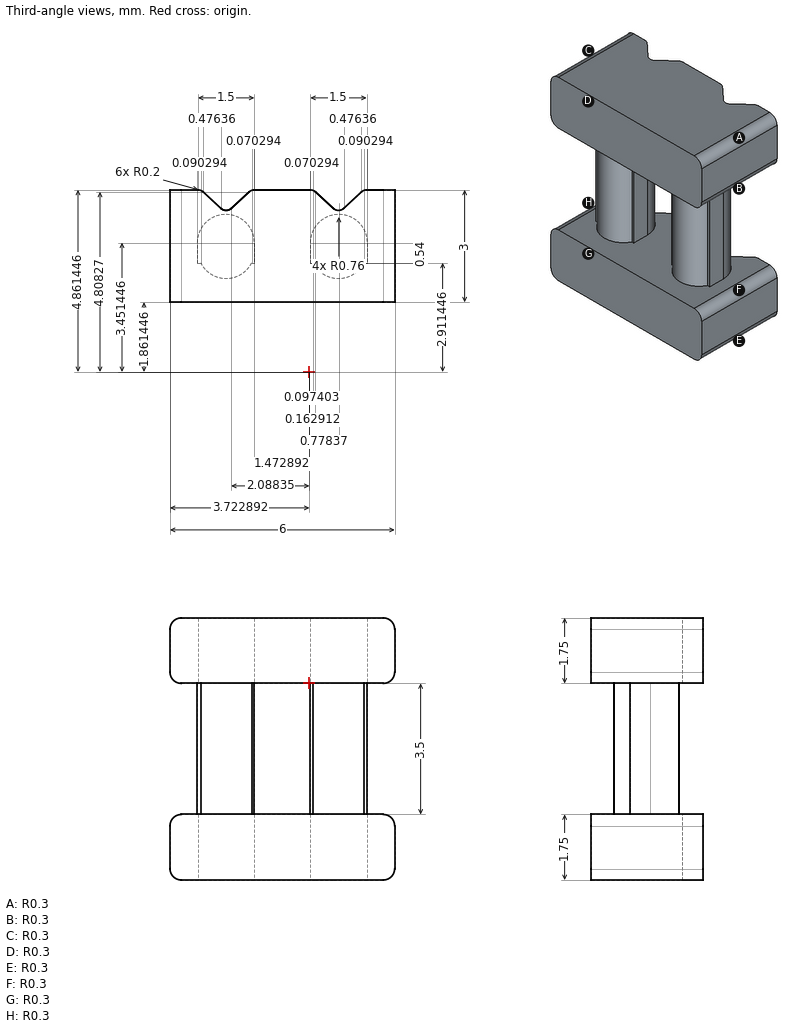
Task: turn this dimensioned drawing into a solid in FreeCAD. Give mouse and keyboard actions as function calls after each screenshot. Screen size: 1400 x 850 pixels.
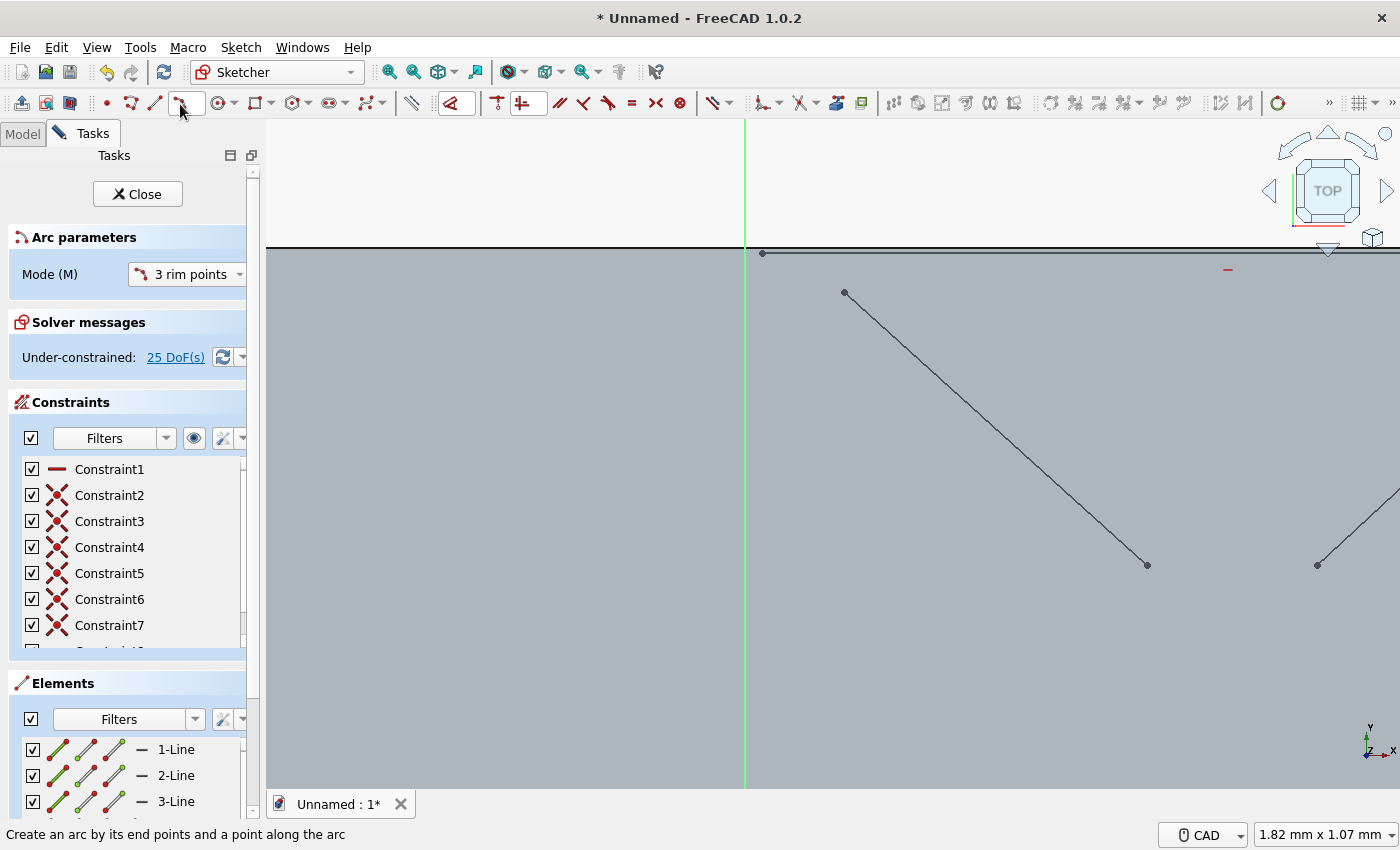
scroll(838, 249, down, 10)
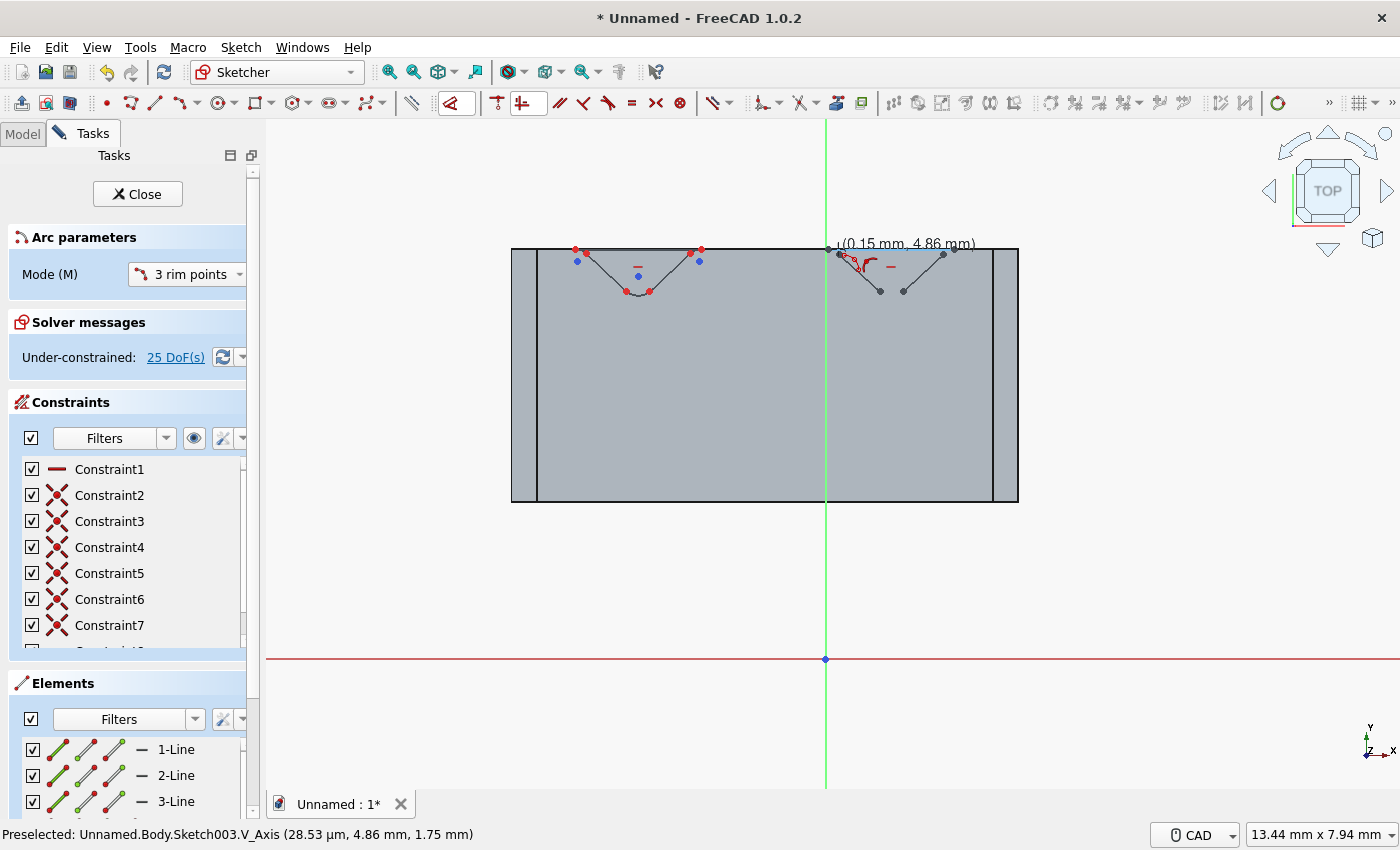
click(880, 292)
click(903, 292)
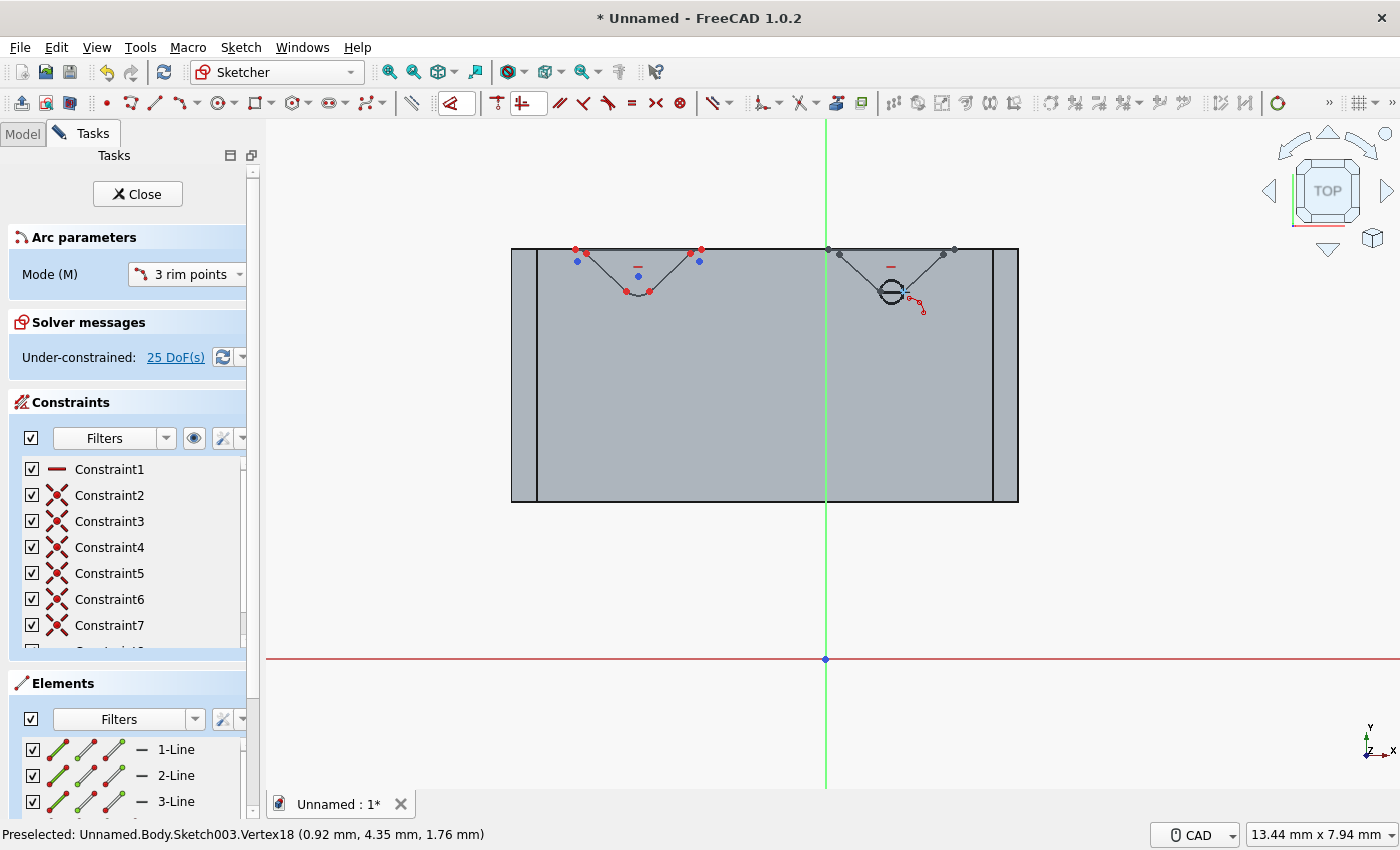
scroll(892, 295, up, 7)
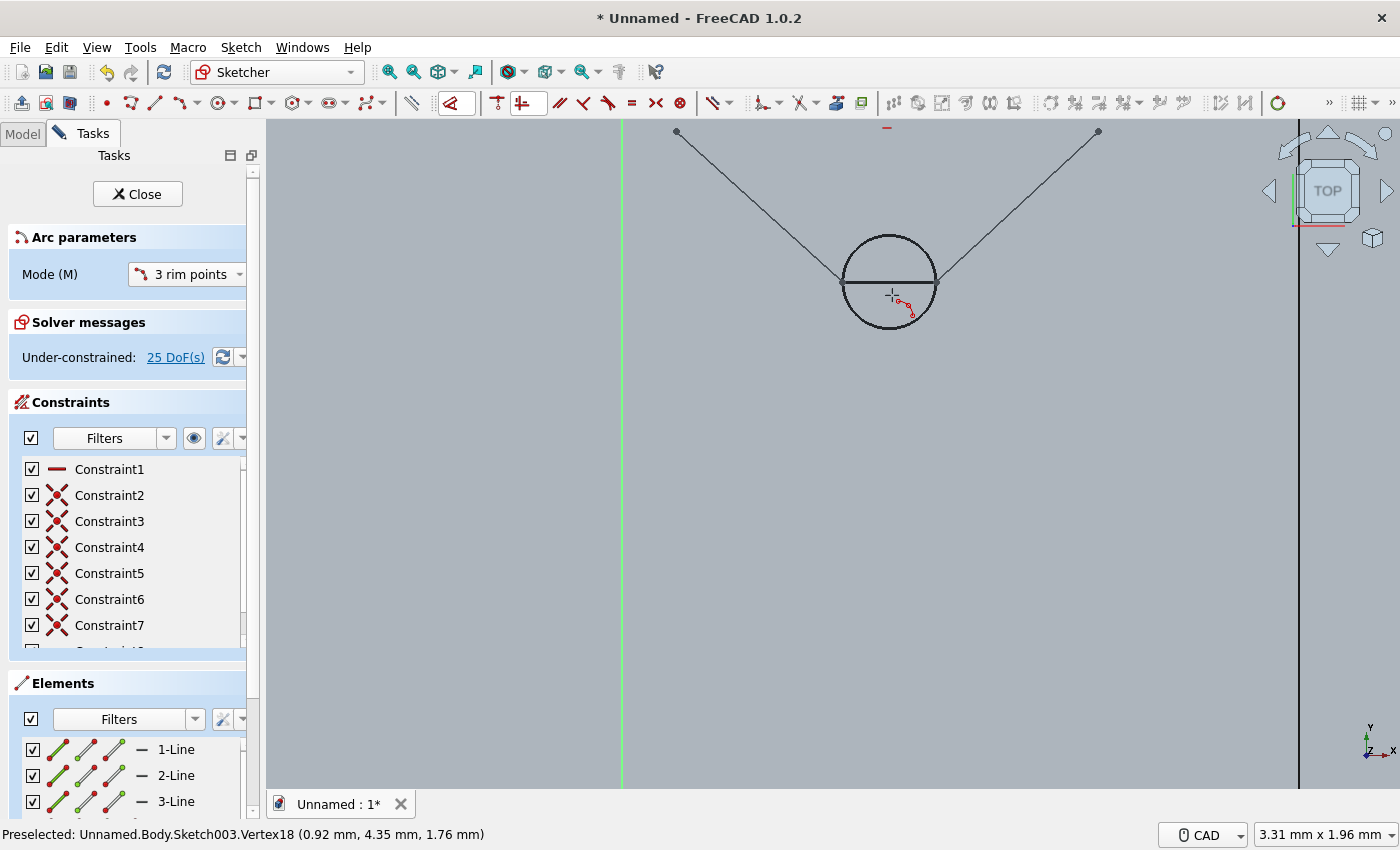
click(889, 296)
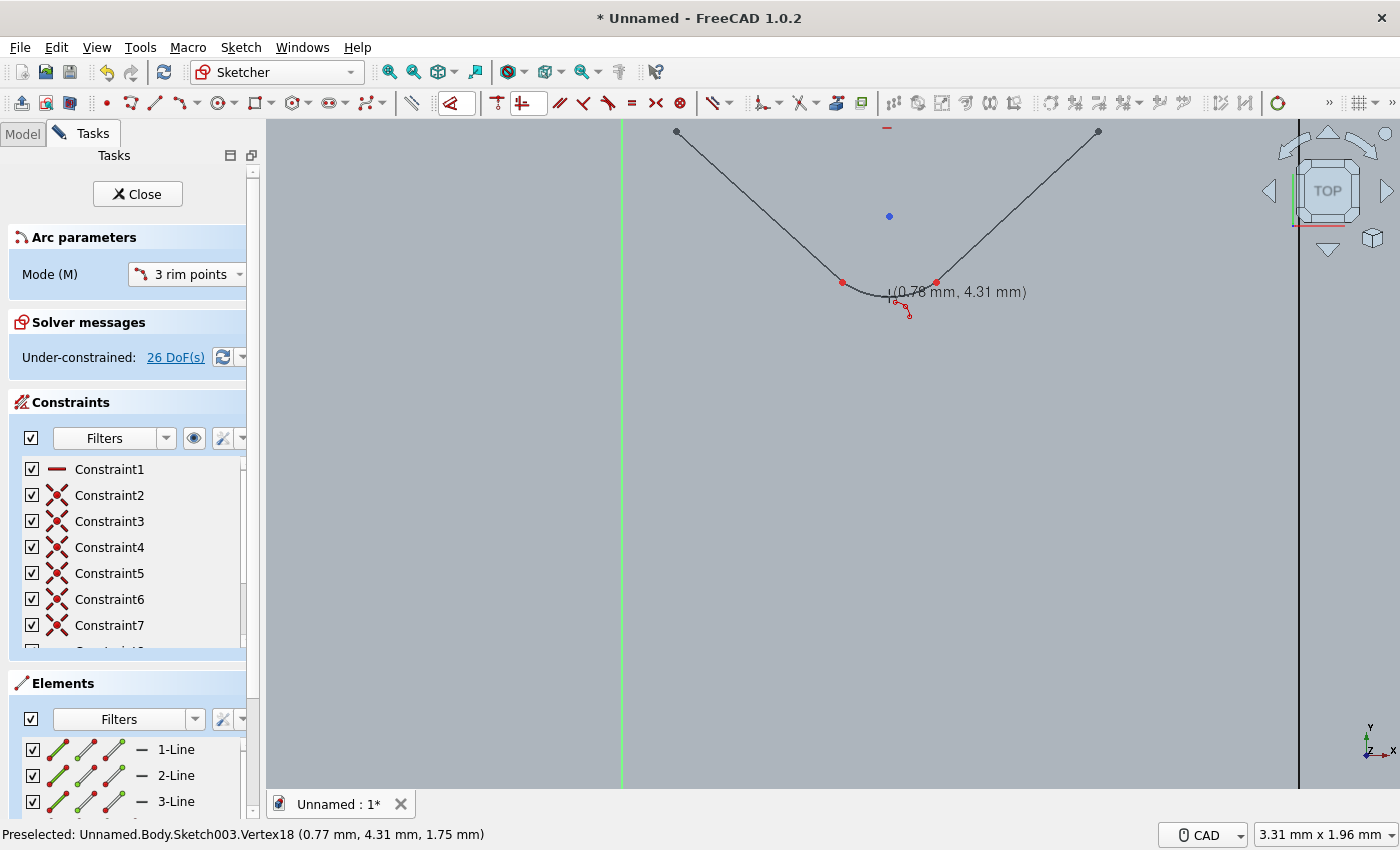
scroll(892, 295, down, 7)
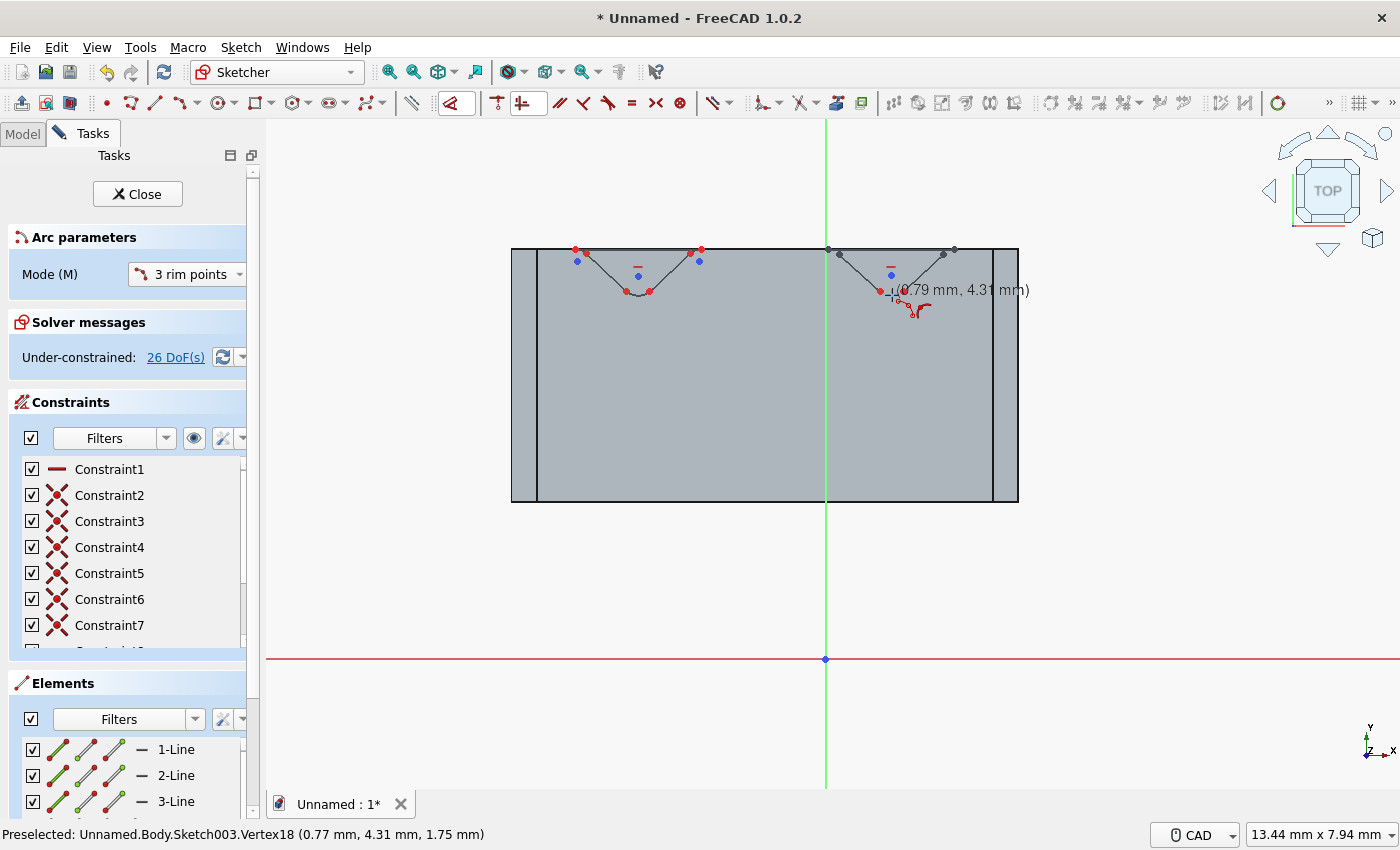
scroll(943, 254, up, 7)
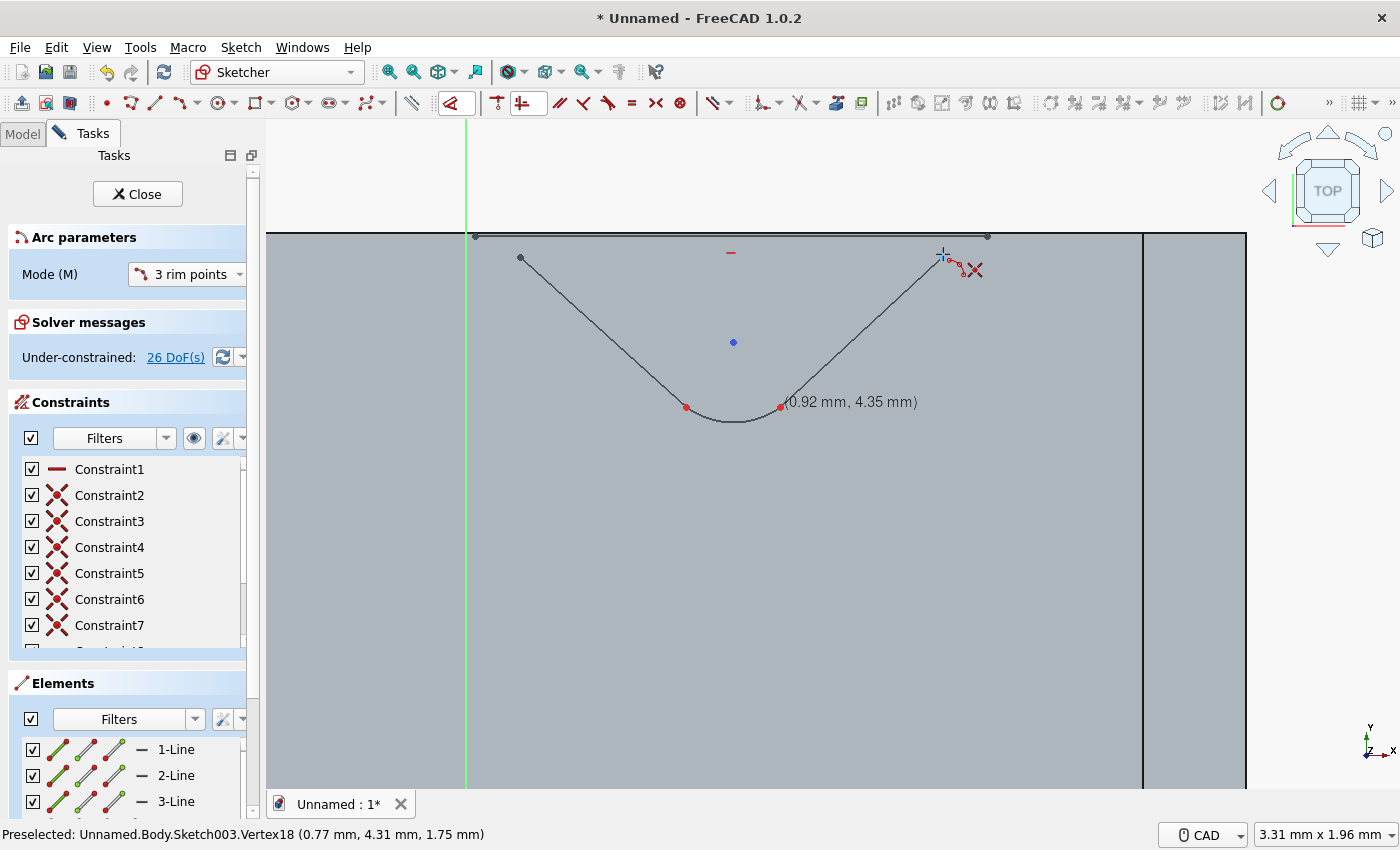
click(942, 257)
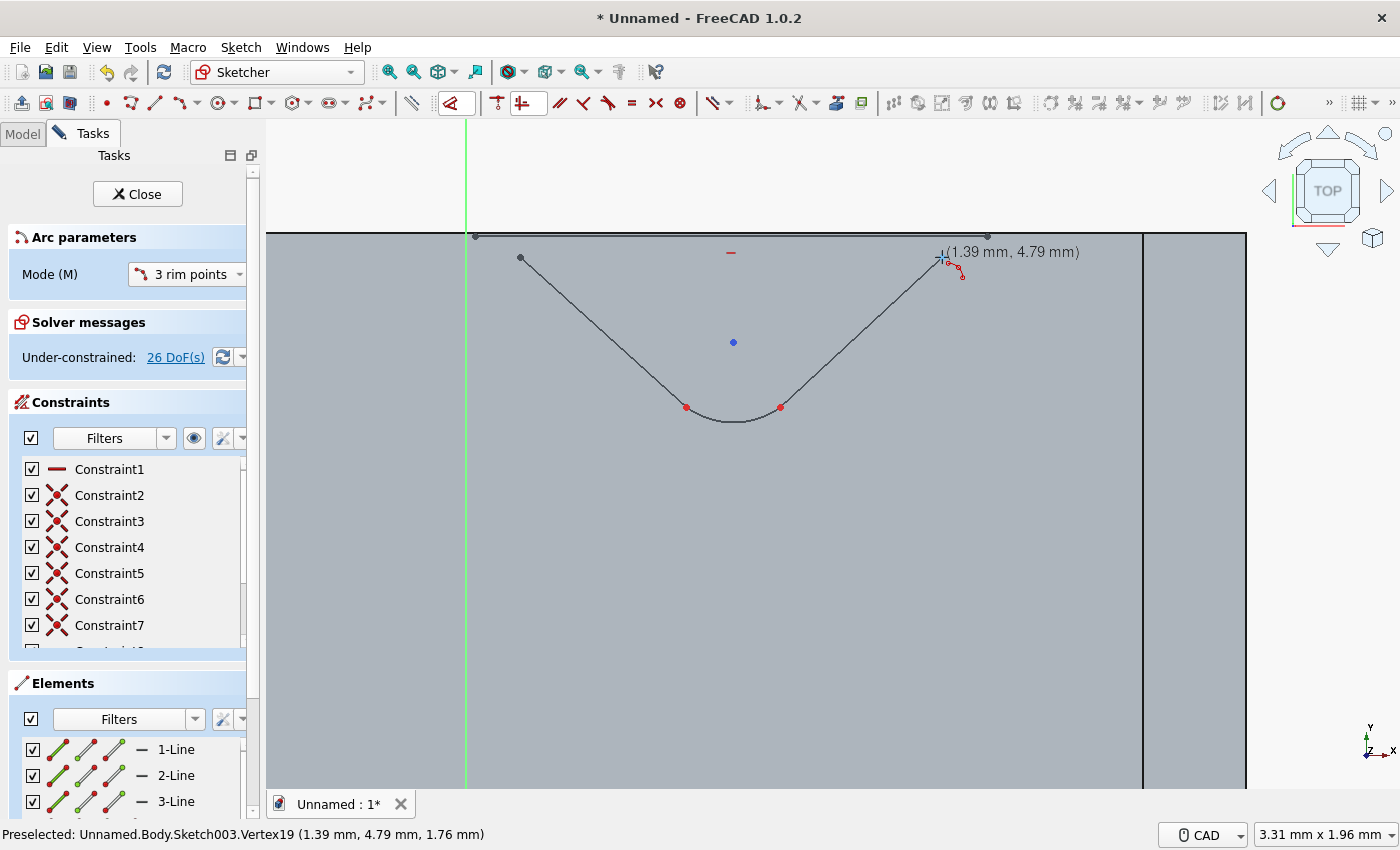
scroll(943, 254, down, 7)